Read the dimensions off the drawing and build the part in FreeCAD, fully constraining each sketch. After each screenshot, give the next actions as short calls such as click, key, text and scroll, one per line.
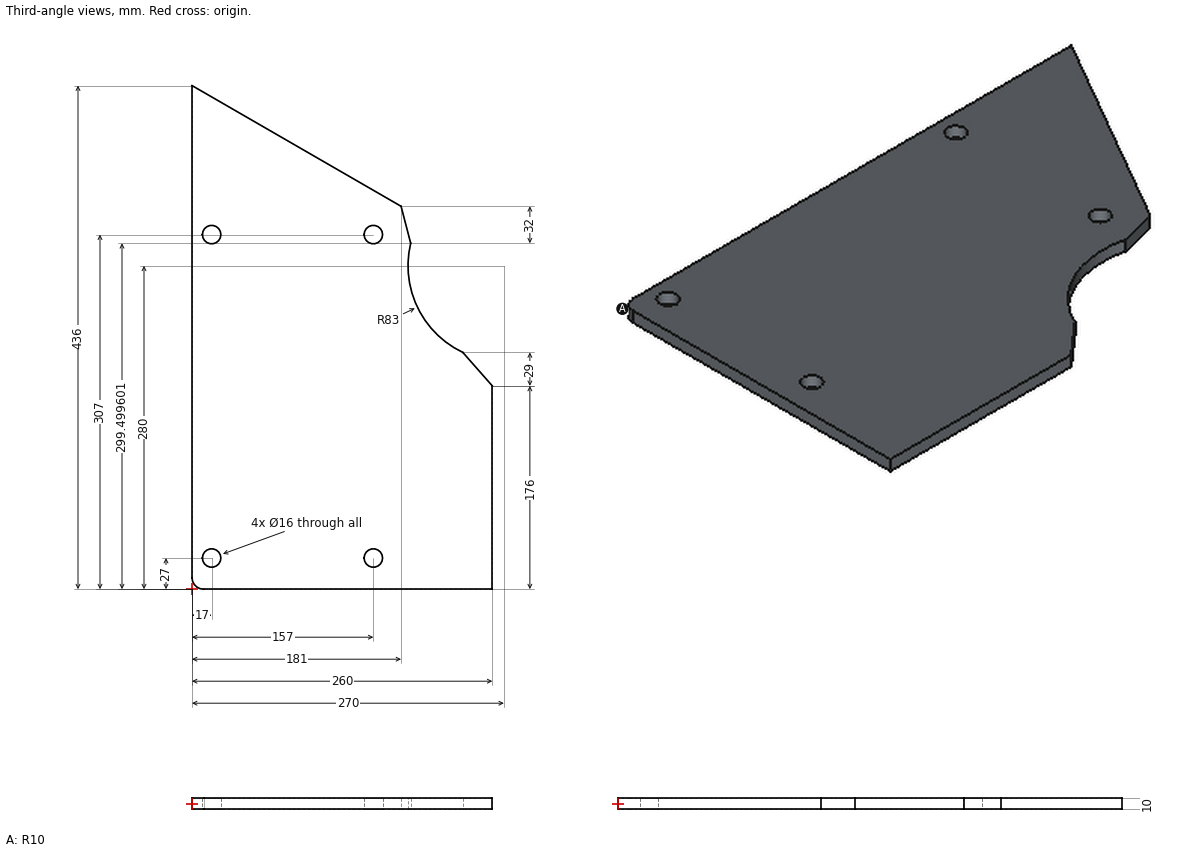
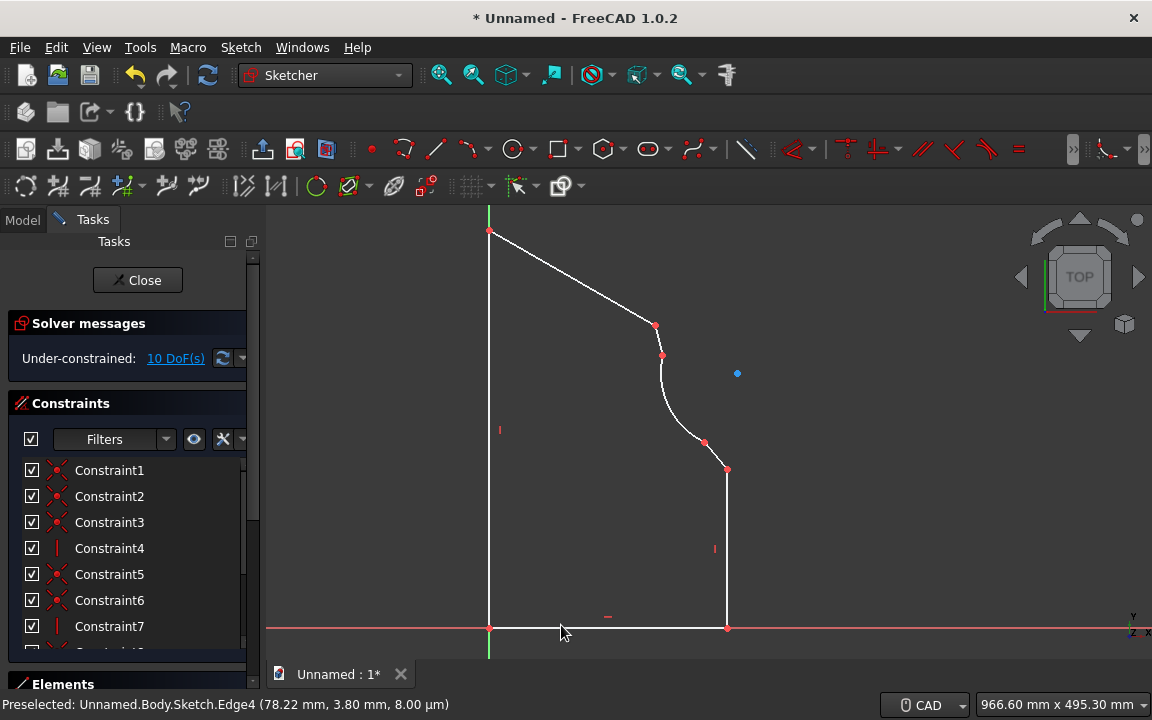
key(d)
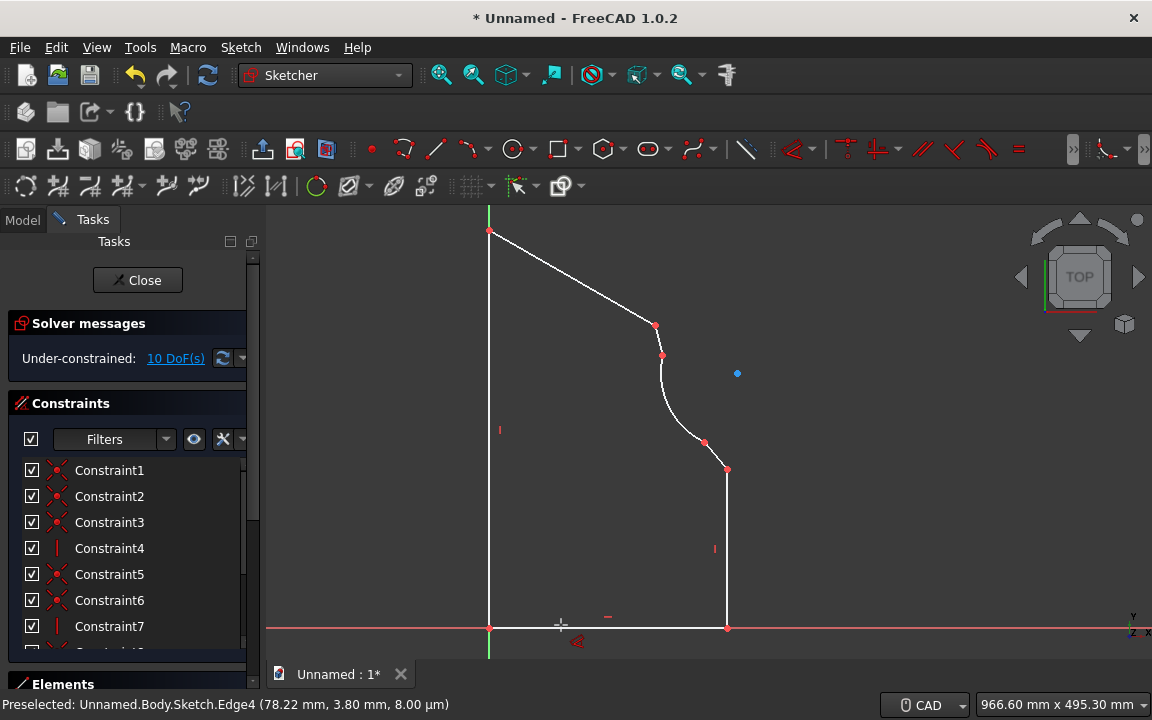
click(662, 387)
click(631, 393)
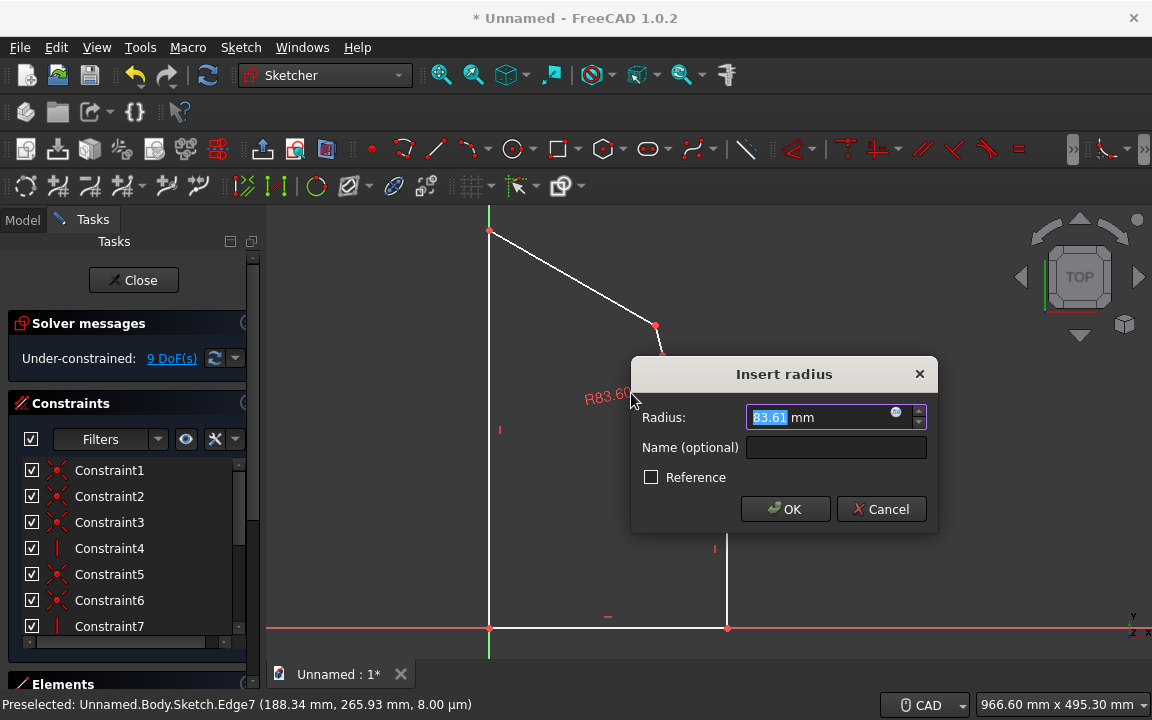
text(83)
key(Return)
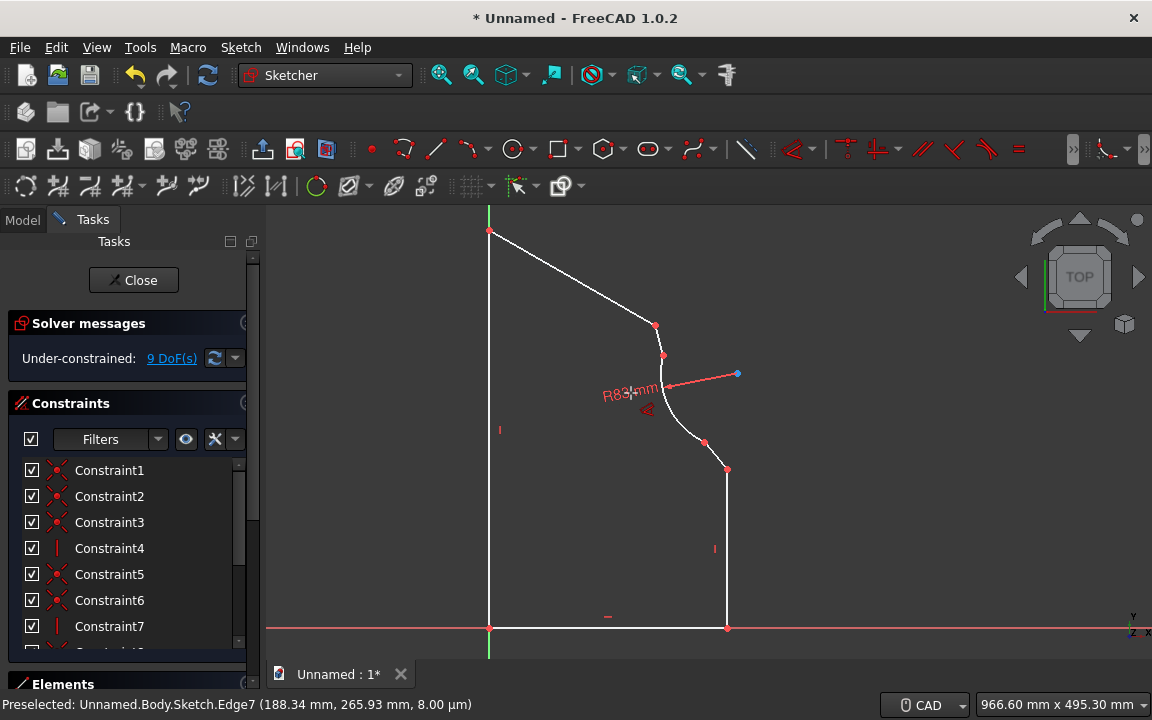
click(489, 350)
click(455, 431)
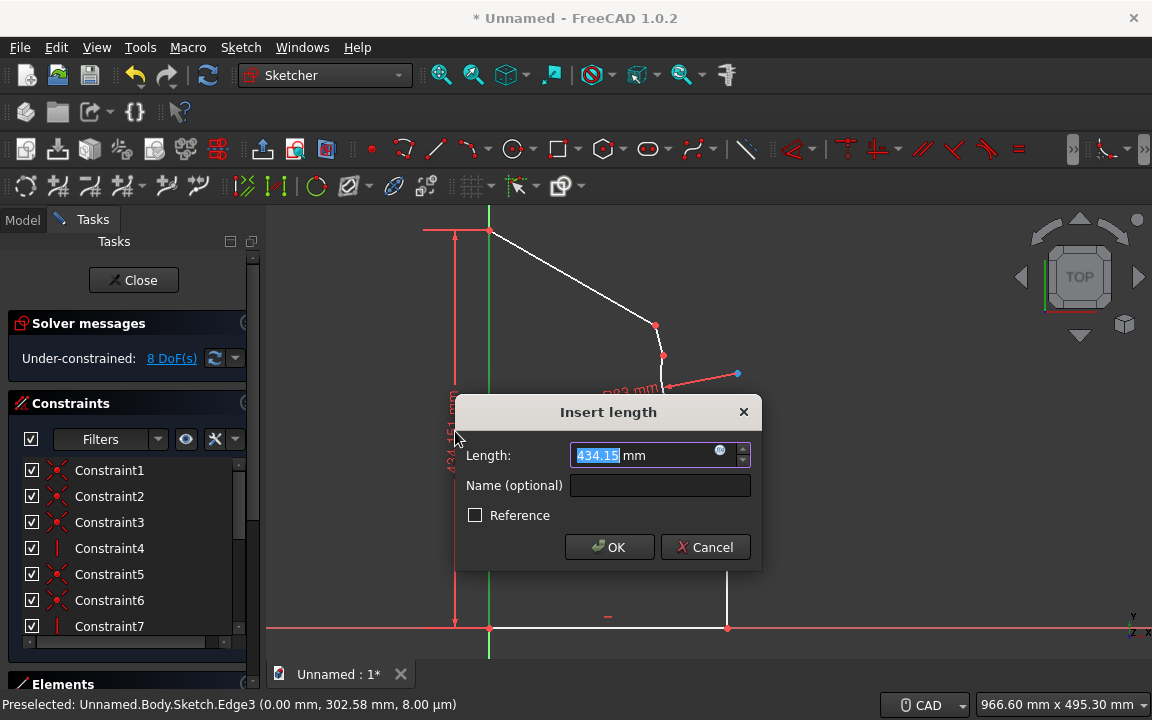
text(436)
key(Return)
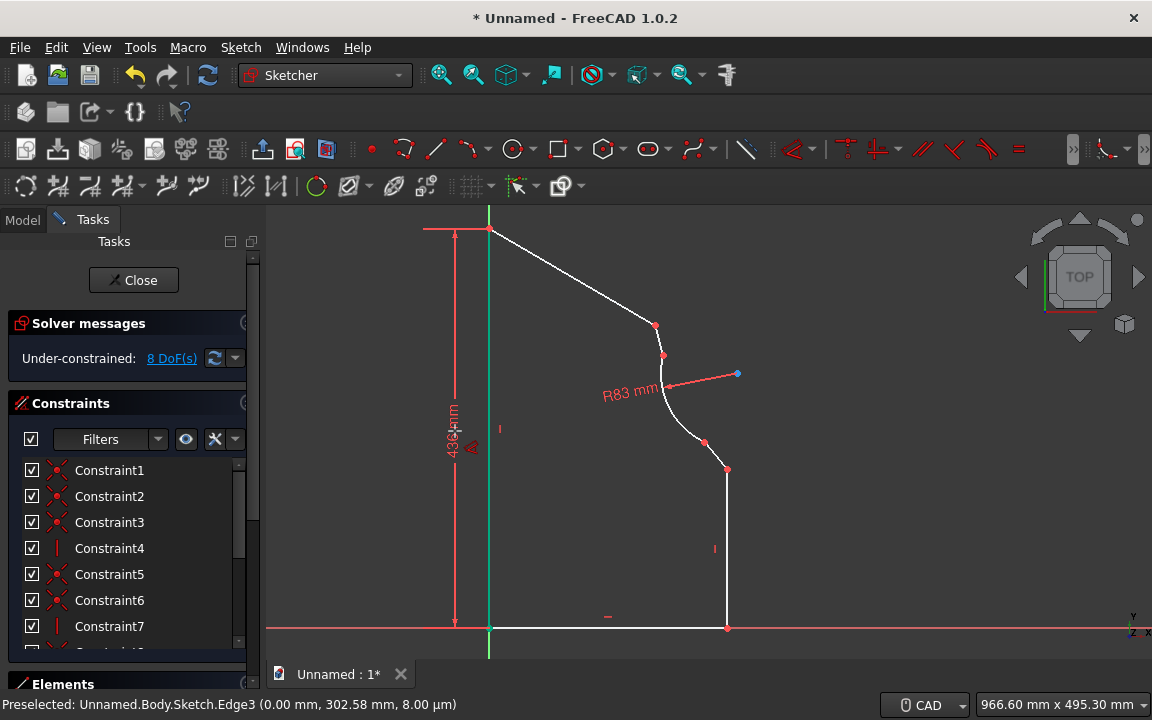
click(561, 628)
click(608, 594)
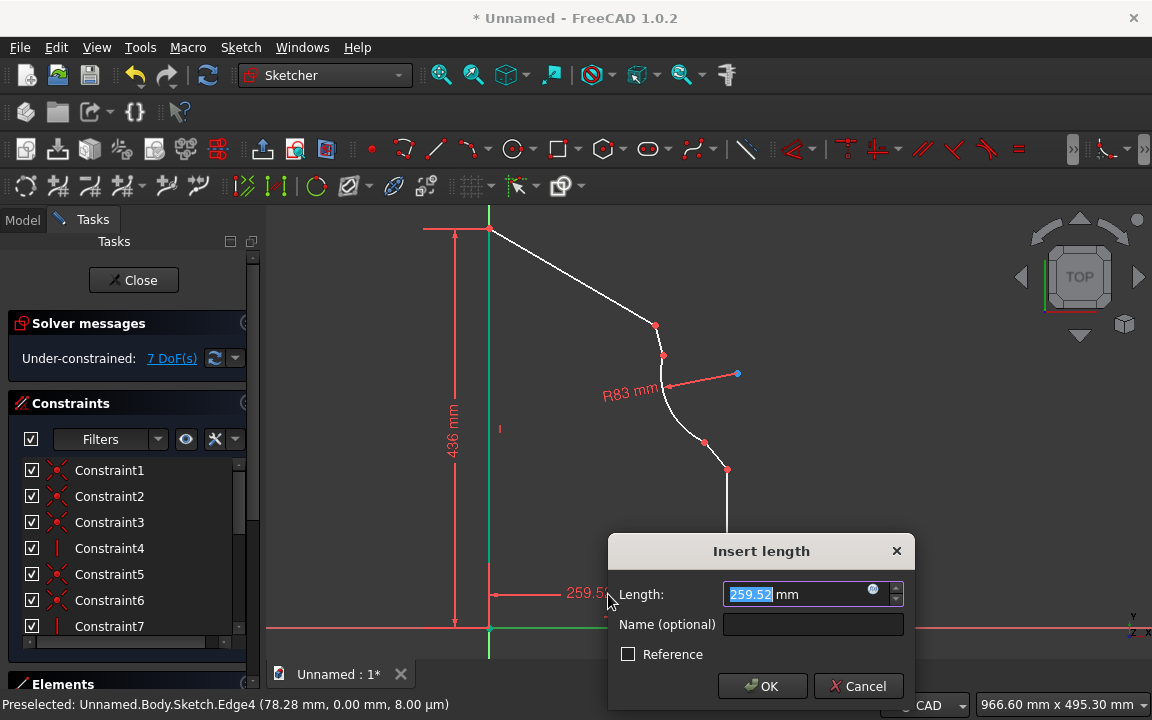
text(260)
key(Return)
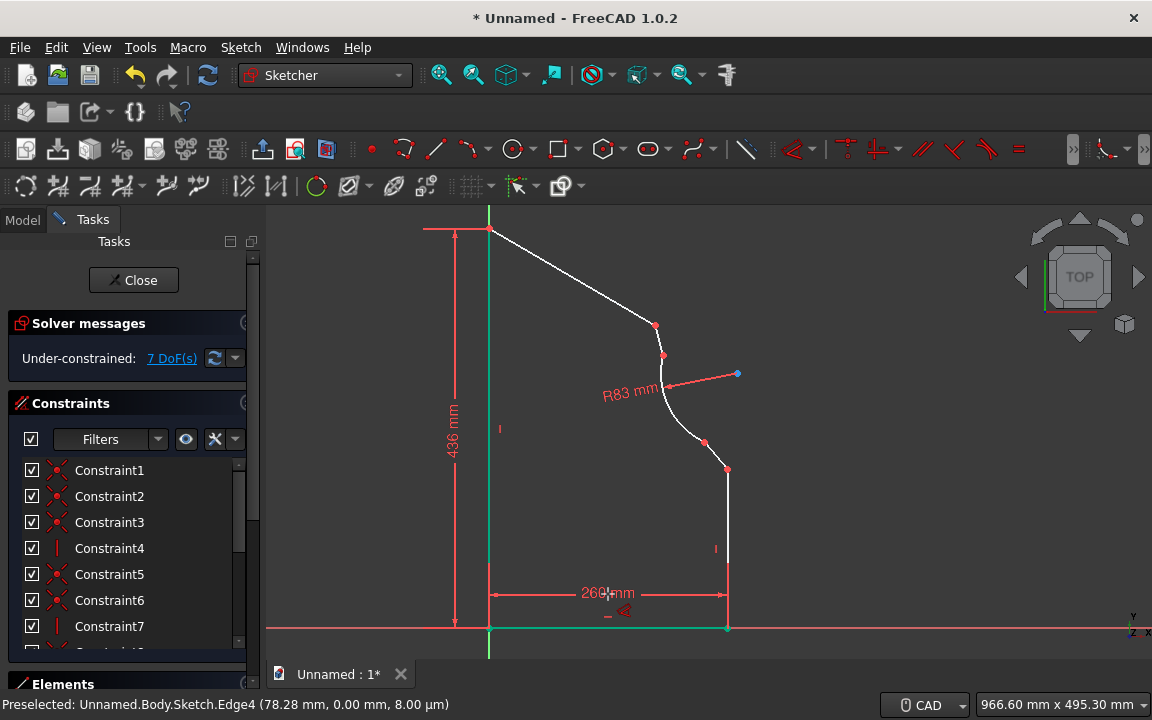
click(728, 581)
click(762, 549)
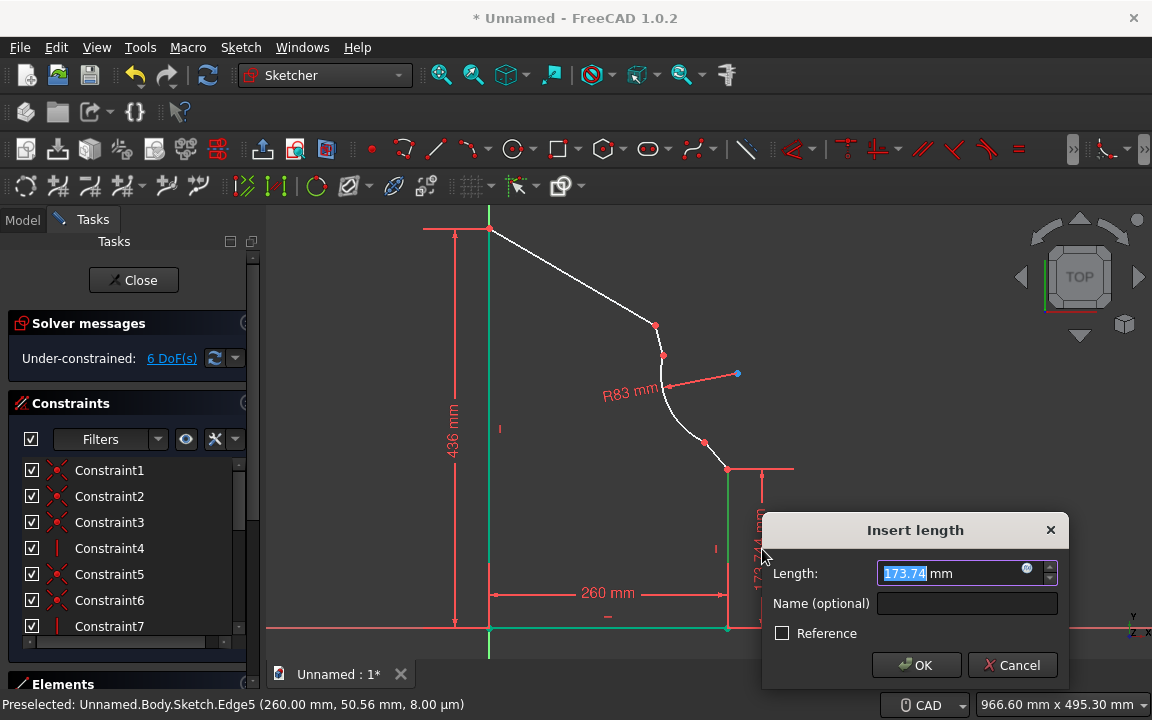
text(176)
key(Return)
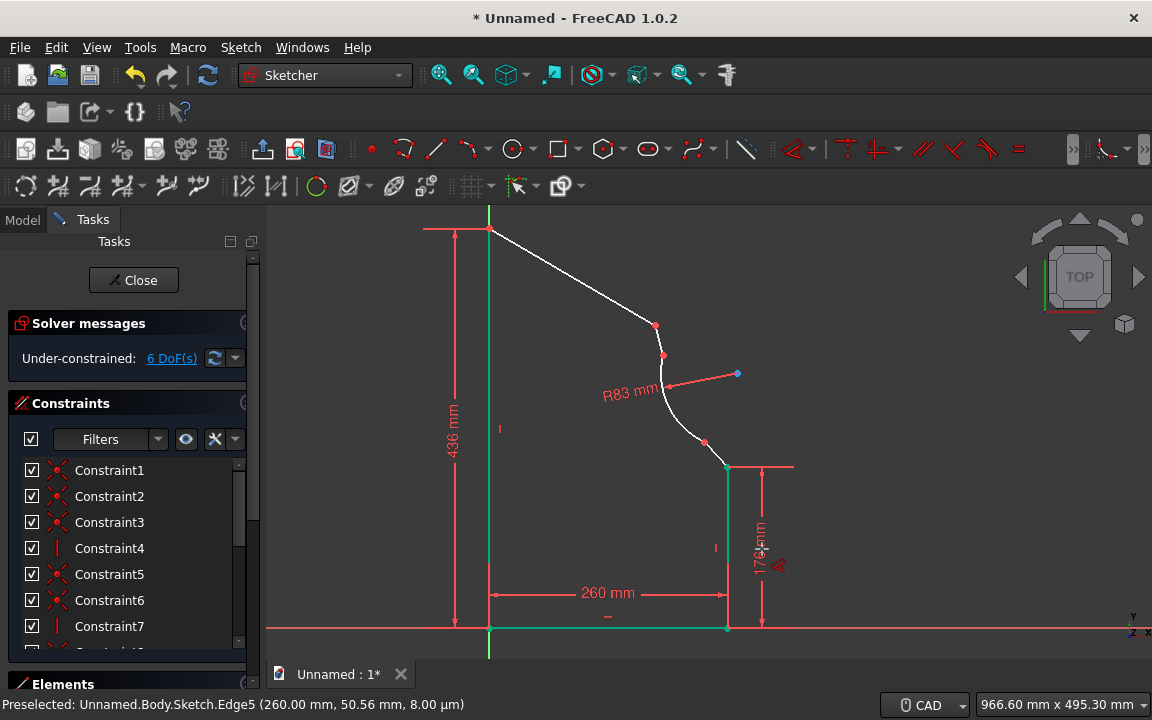
scroll(661, 347, up, 3)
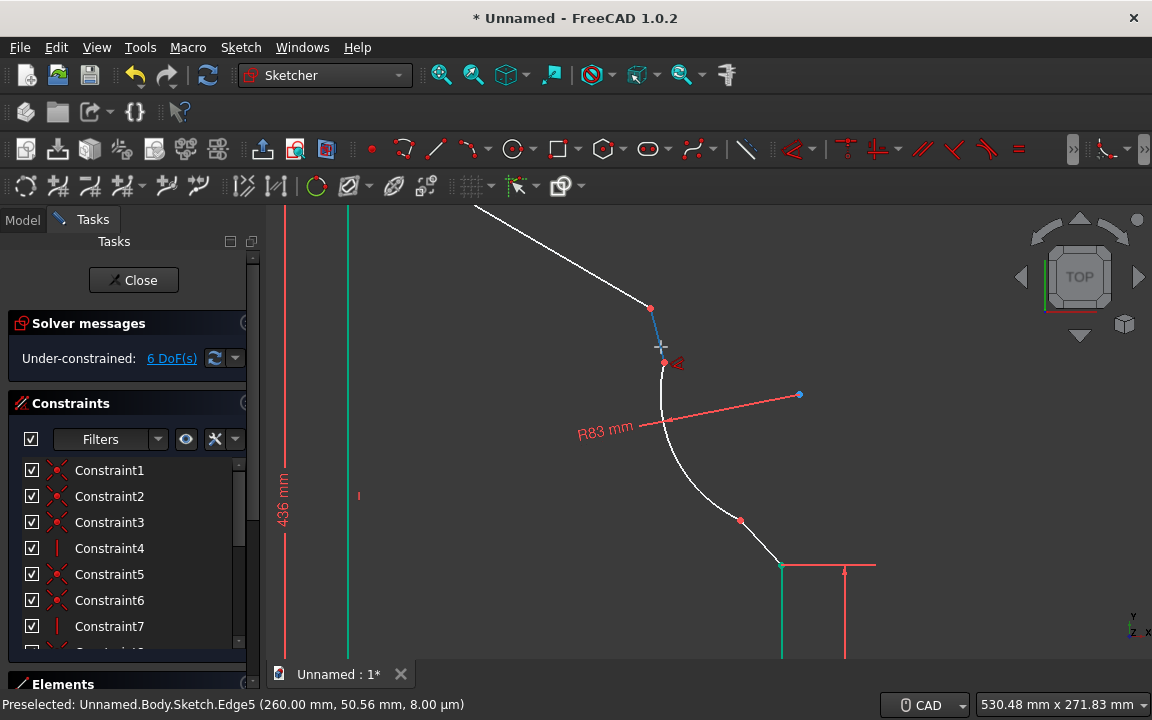
click(660, 346)
click(698, 335)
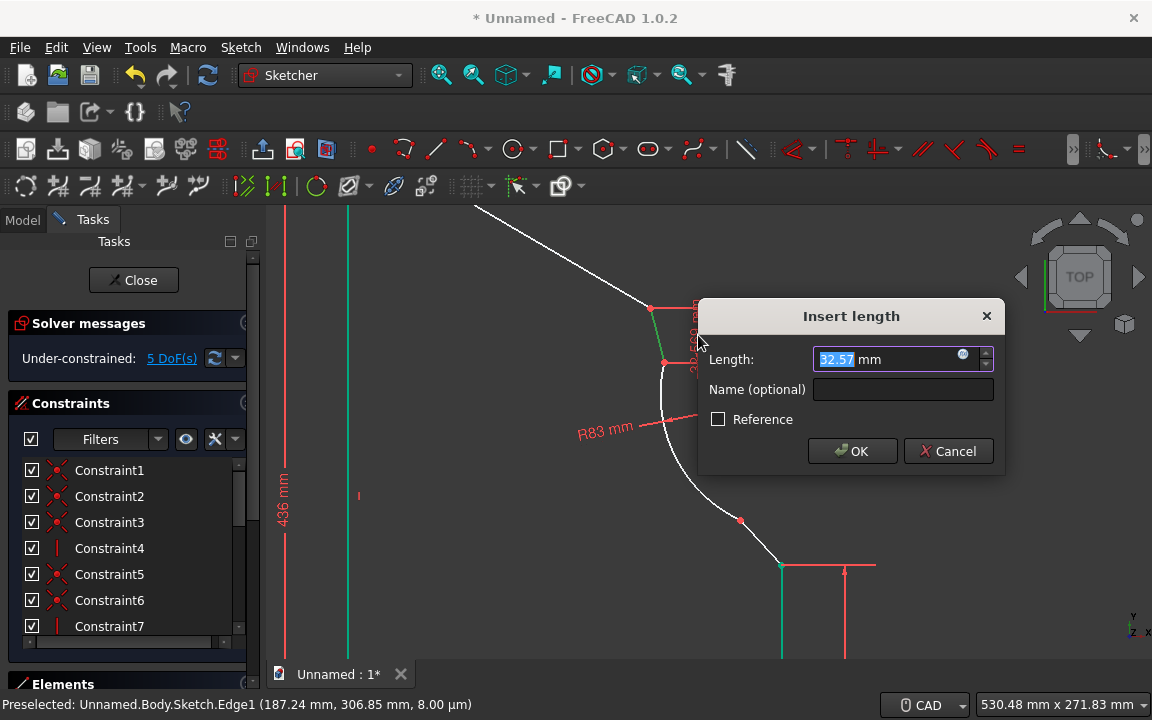
text(32)
key(Return)